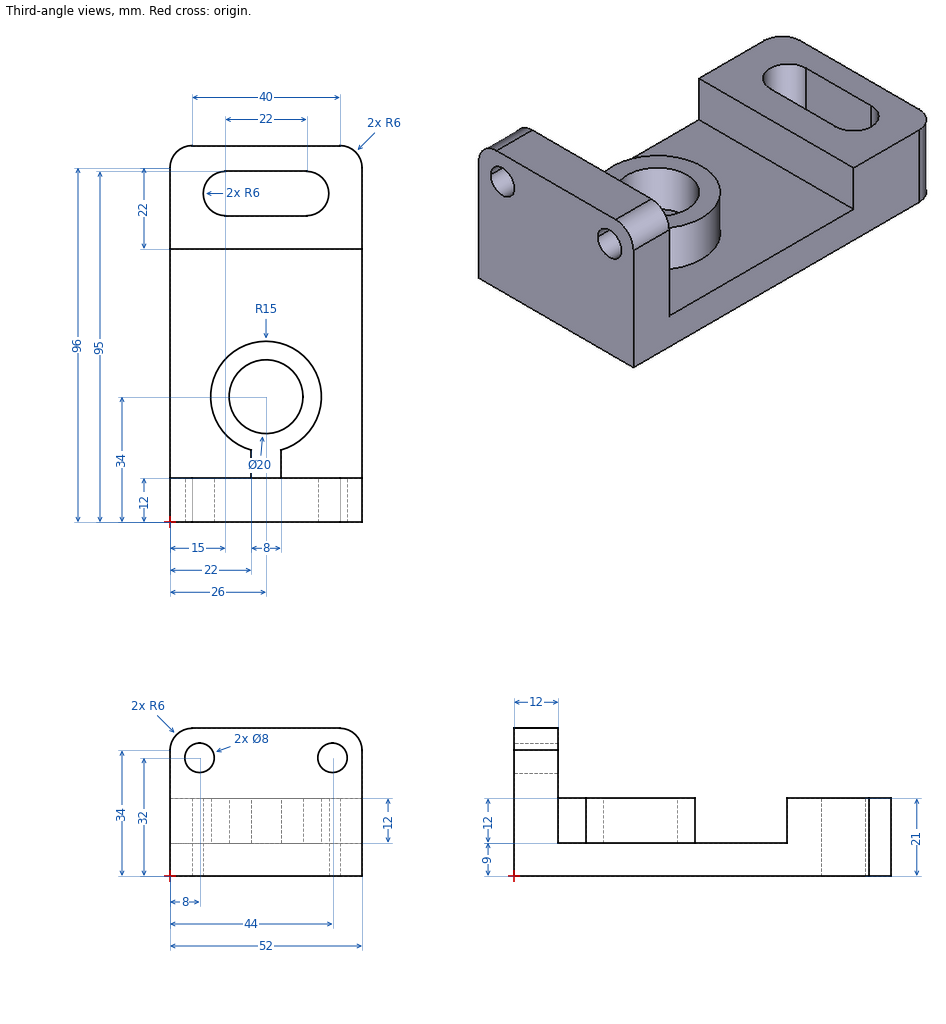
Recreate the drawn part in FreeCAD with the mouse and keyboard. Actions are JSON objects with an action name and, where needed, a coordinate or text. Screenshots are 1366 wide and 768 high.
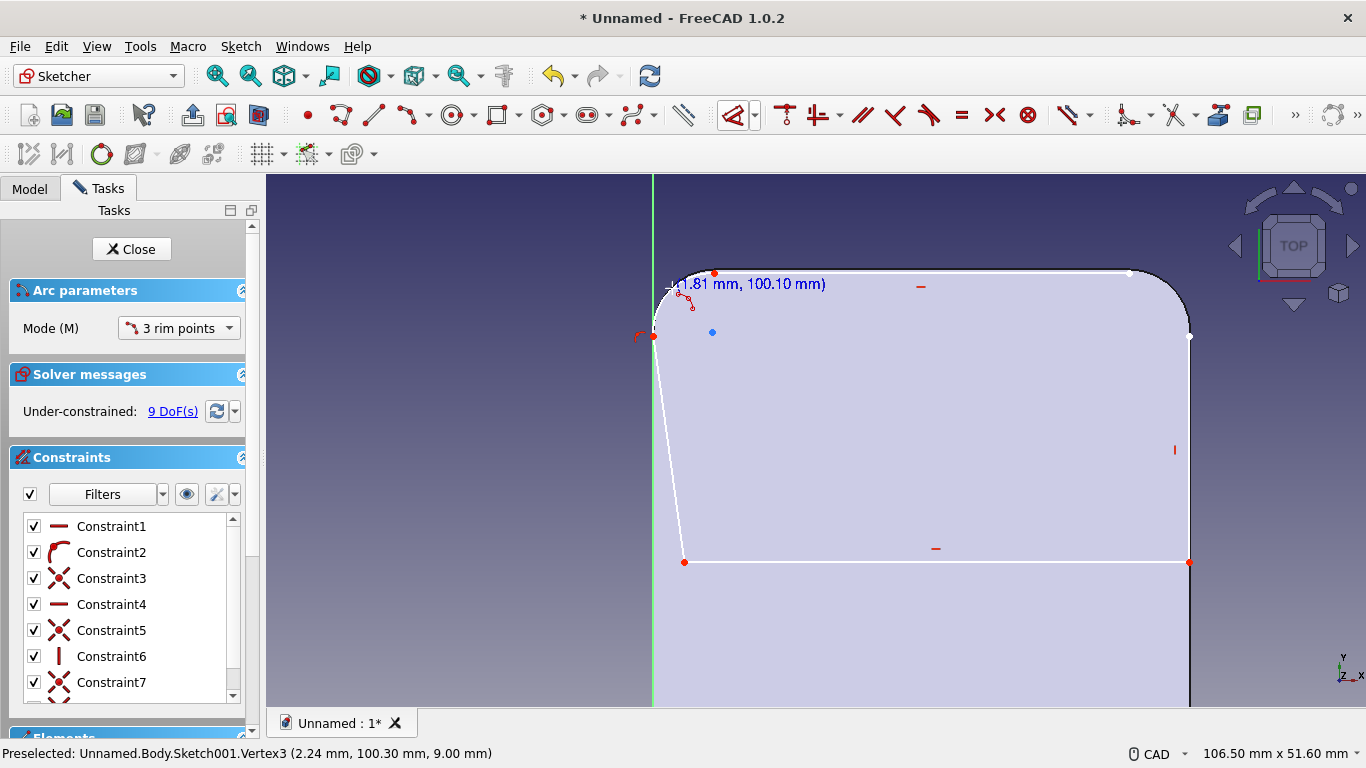
{"action": "left_click", "coordinate": [1189, 336]}
{"action": "left_click", "coordinate": [1129, 273]}
{"action": "left_click", "coordinate": [1172, 288]}
{"action": "key", "text": "Escape"}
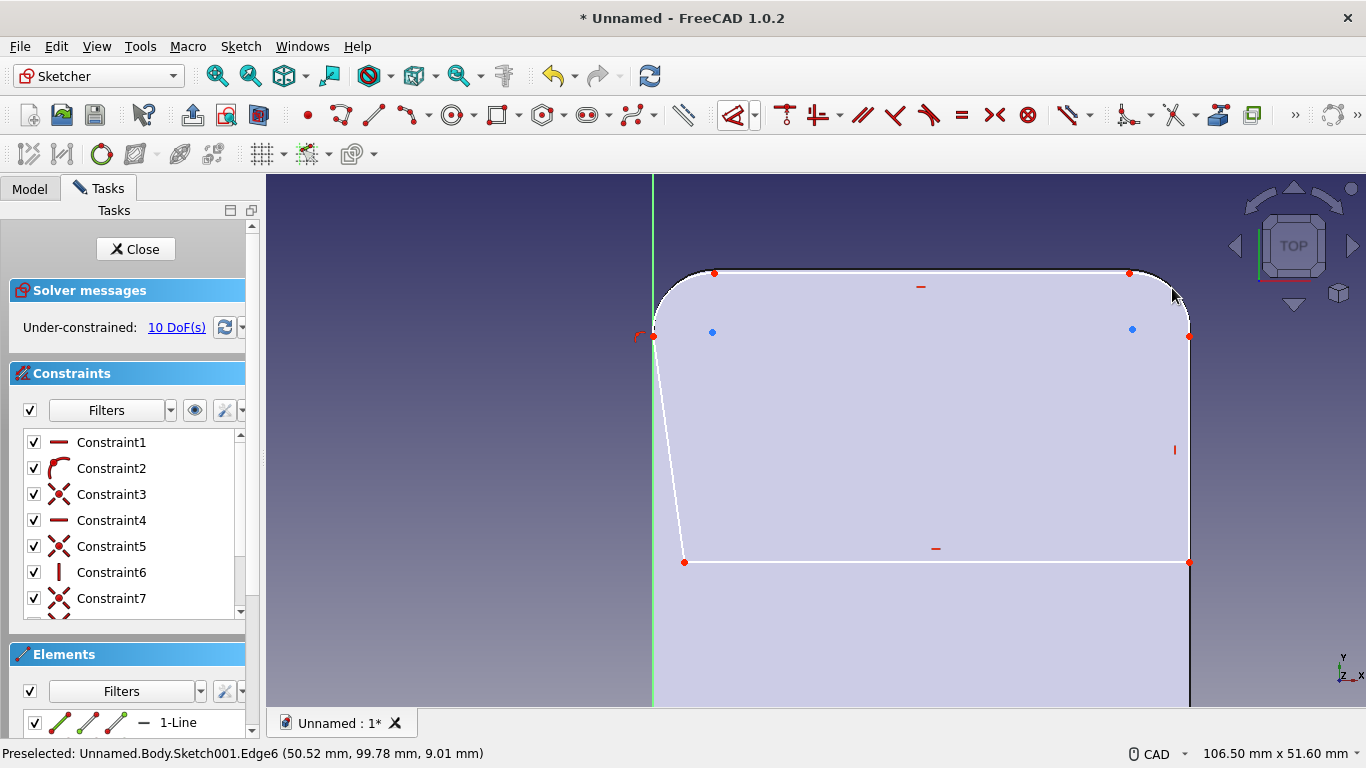
{"action": "left_click", "coordinate": [1005, 273]}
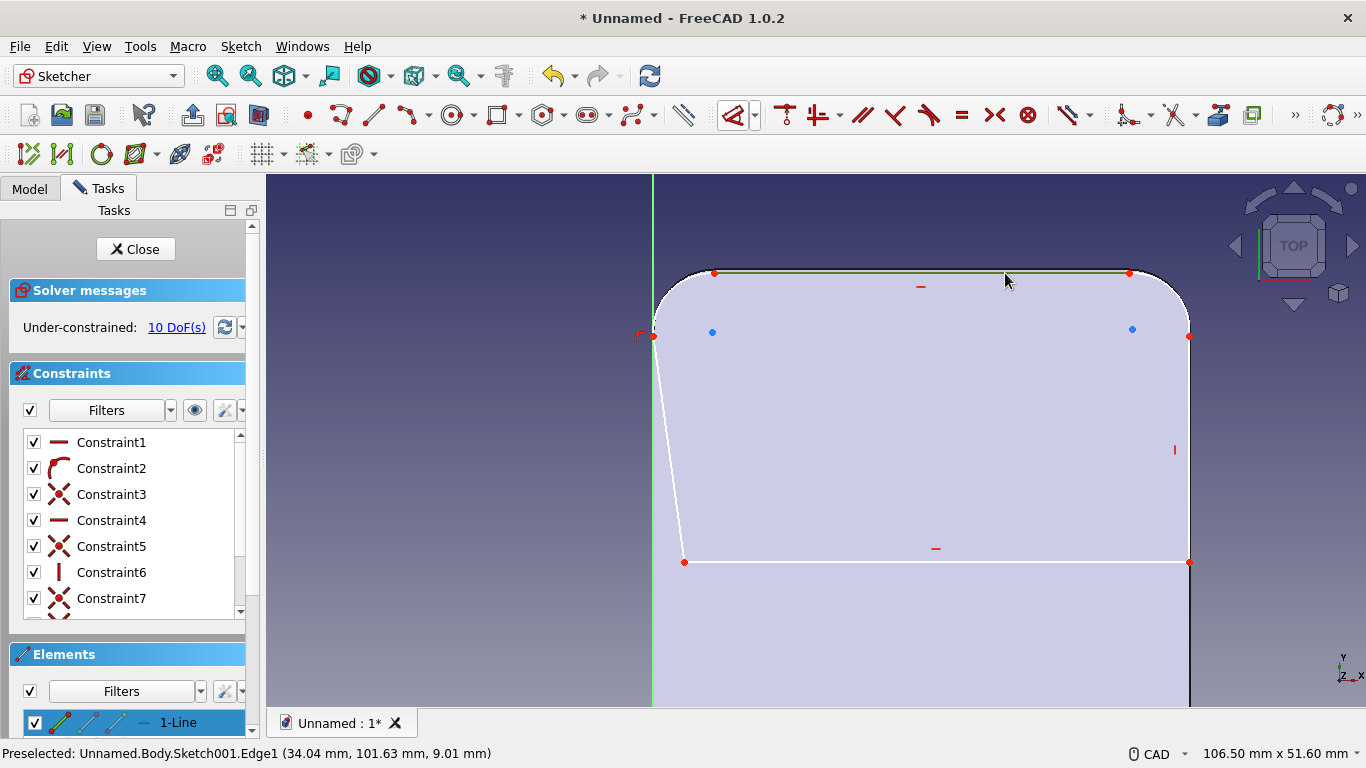
{"action": "left_click", "coordinate": [686, 280]}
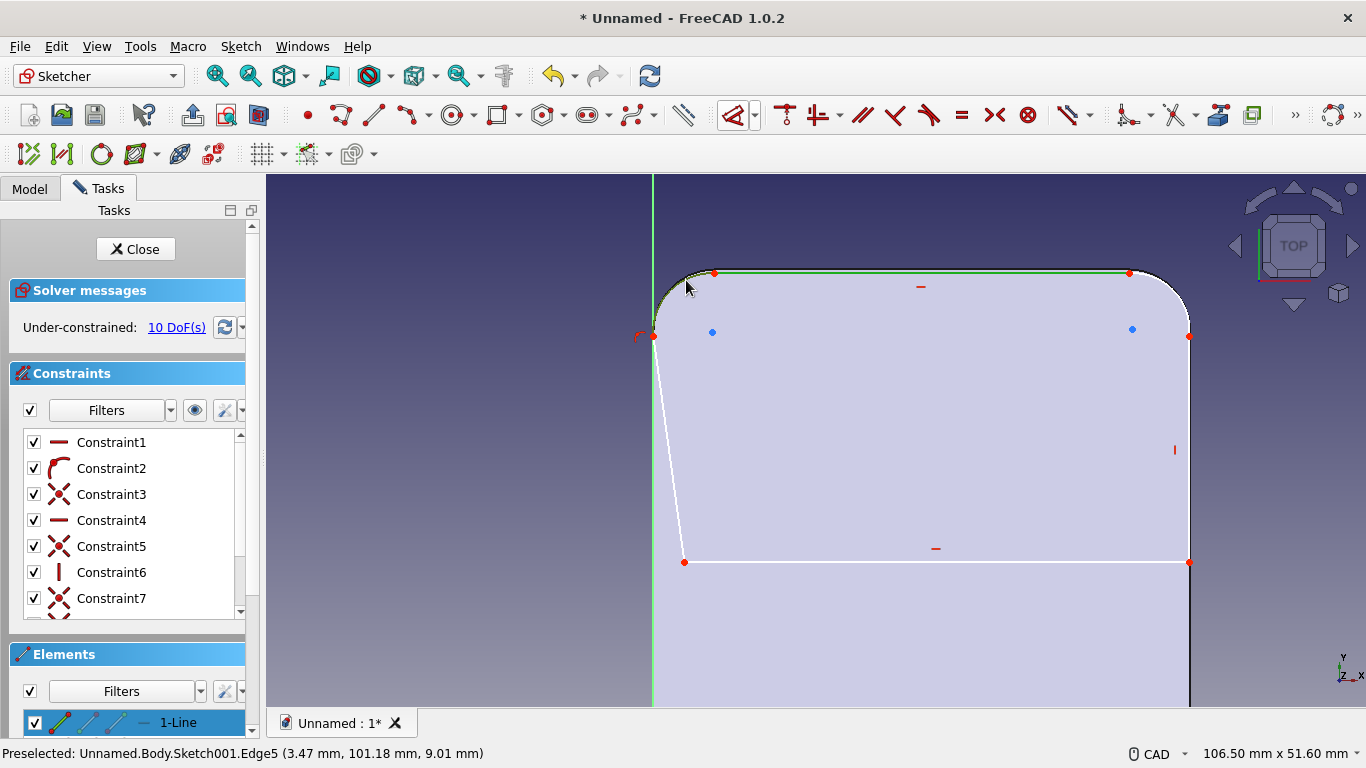
{"action": "left_click", "coordinate": [929, 116]}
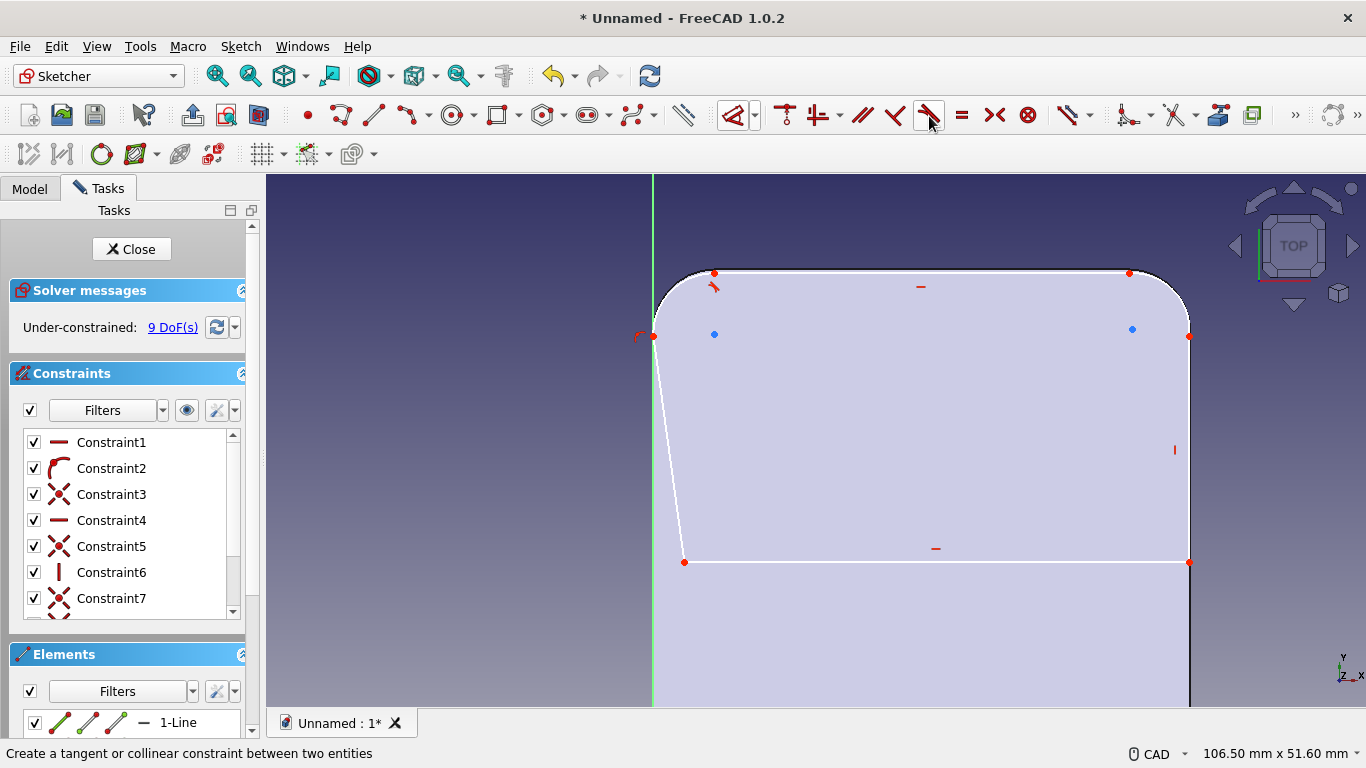
{"action": "left_click", "coordinate": [1005, 273]}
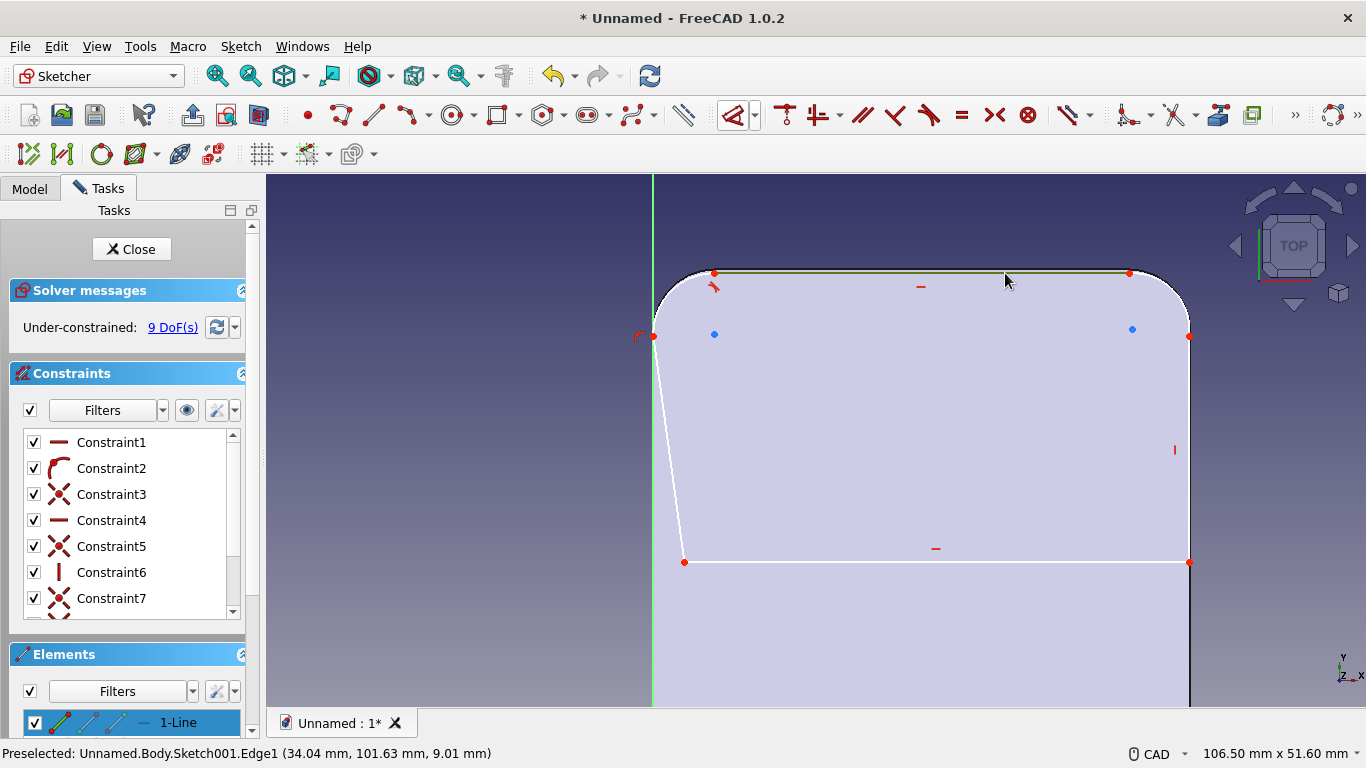
{"action": "left_click", "coordinate": [1185, 307]}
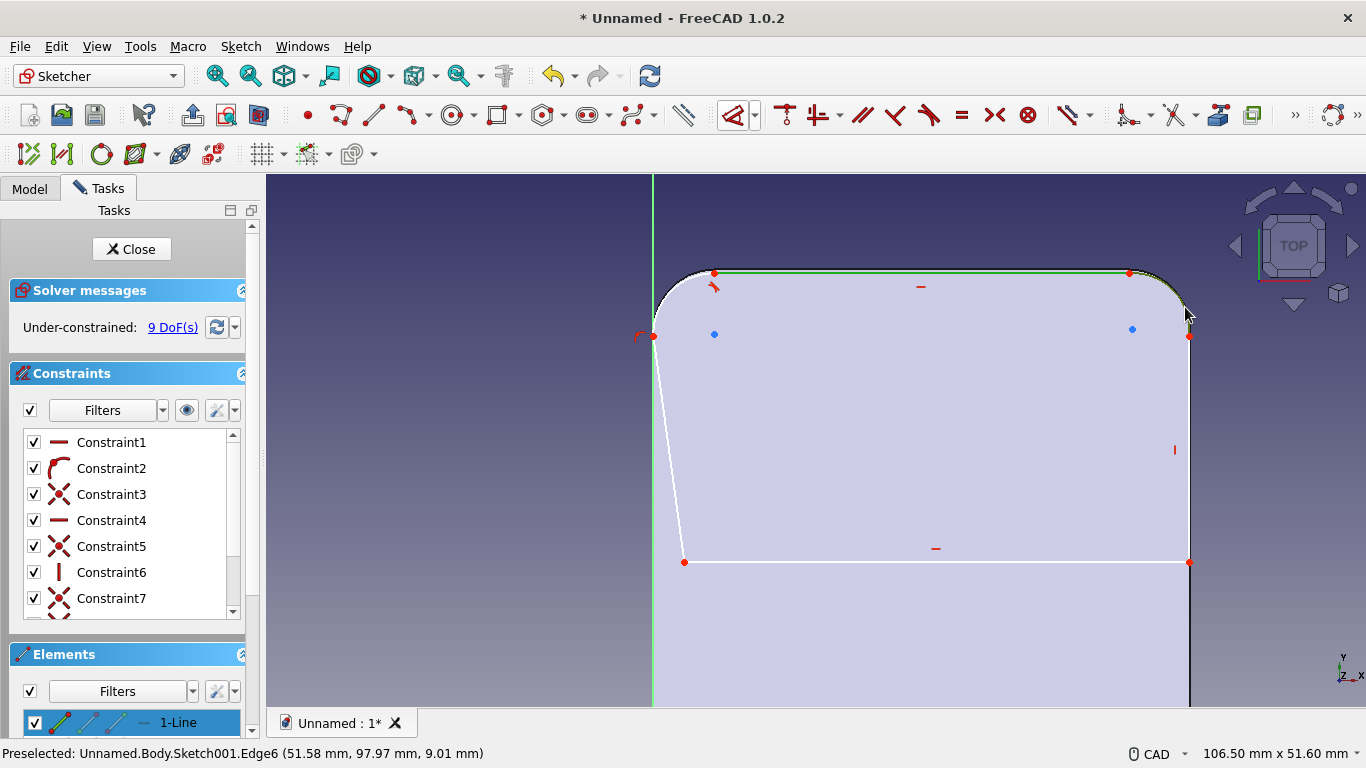
{"action": "key", "text": "t"}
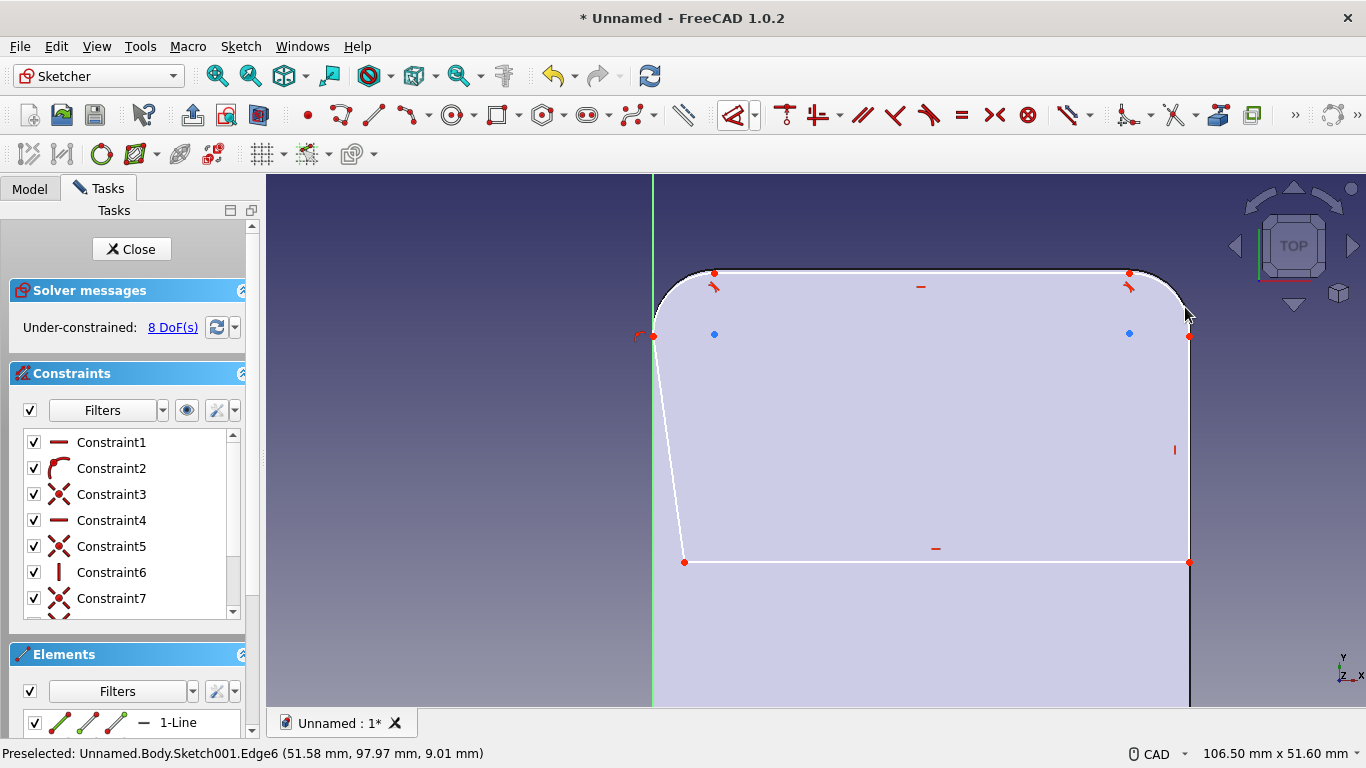
{"action": "scroll", "coordinate": [663, 404], "scroll_direction": "up", "scroll_amount": 2}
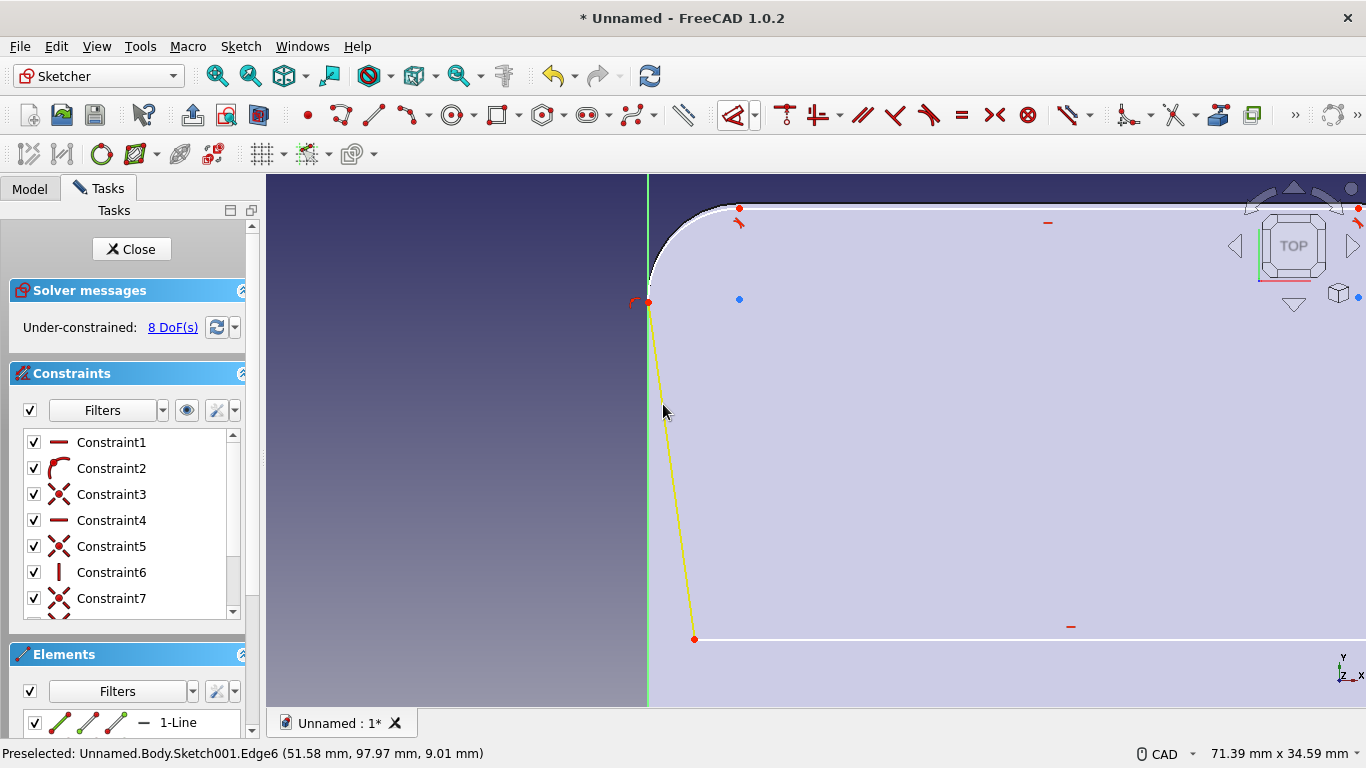
{"action": "left_click", "coordinate": [662, 404]}